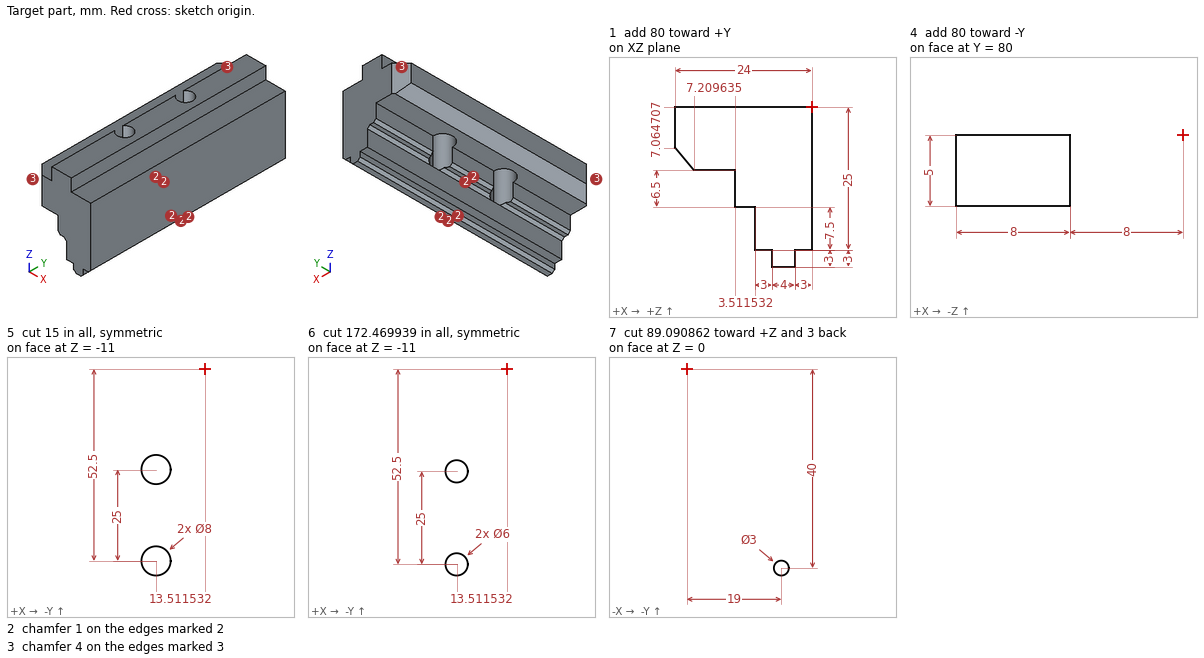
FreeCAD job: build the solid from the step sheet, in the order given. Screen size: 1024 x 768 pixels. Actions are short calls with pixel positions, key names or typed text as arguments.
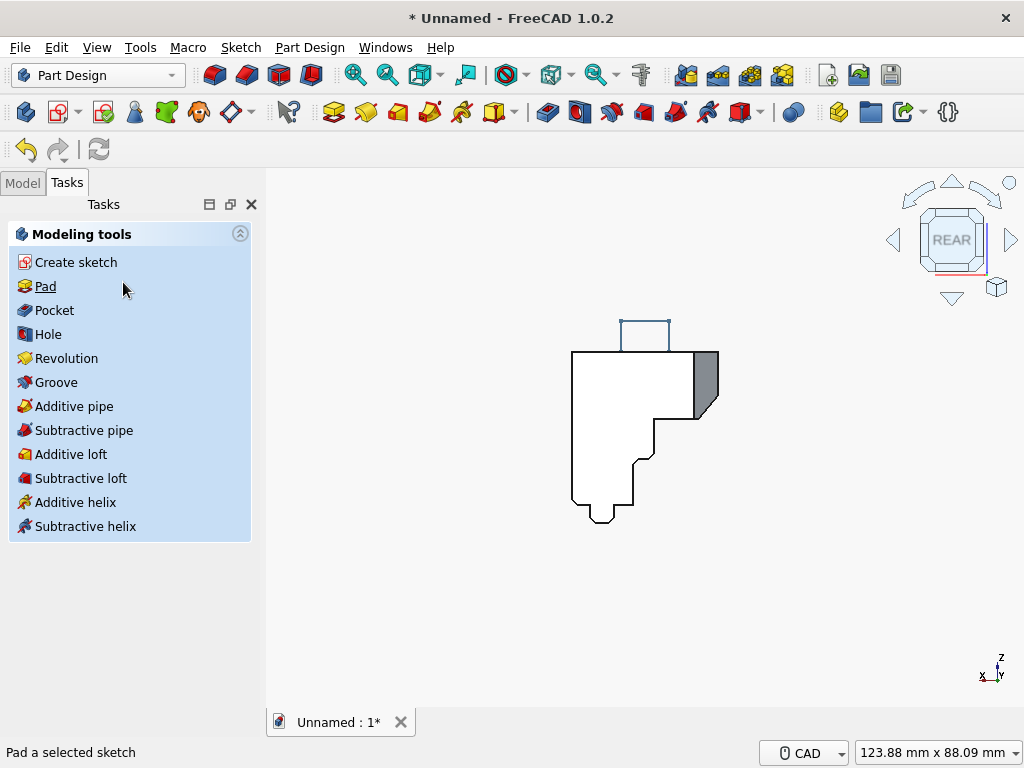
click(334, 112)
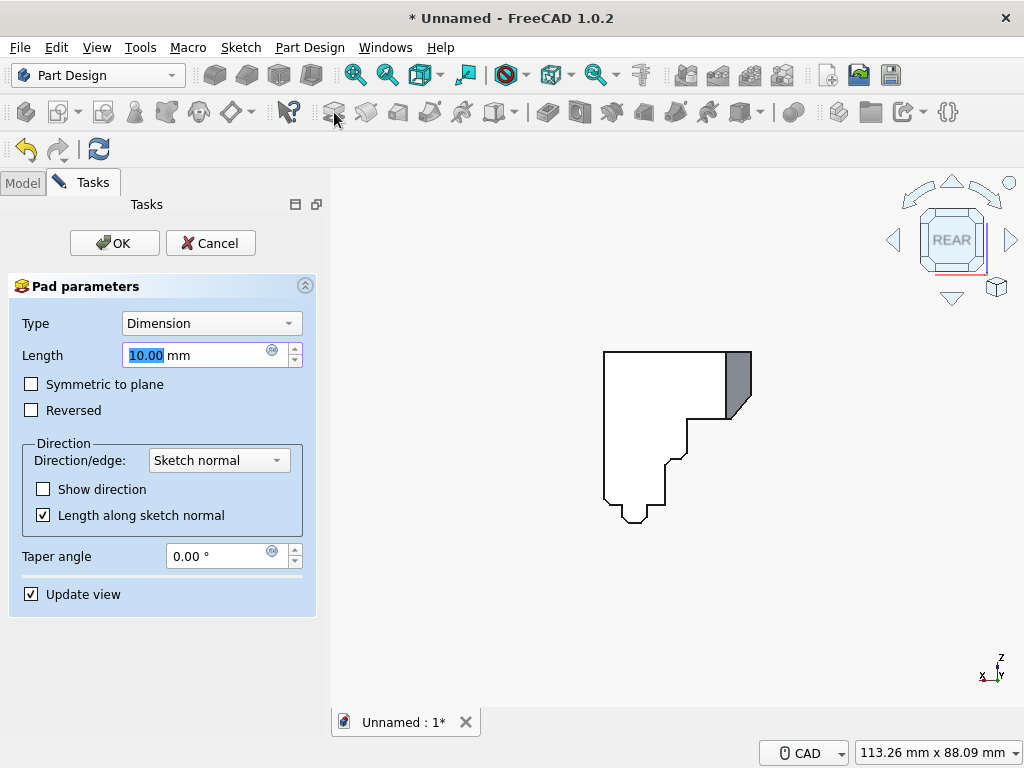
text(80)
key(Tab)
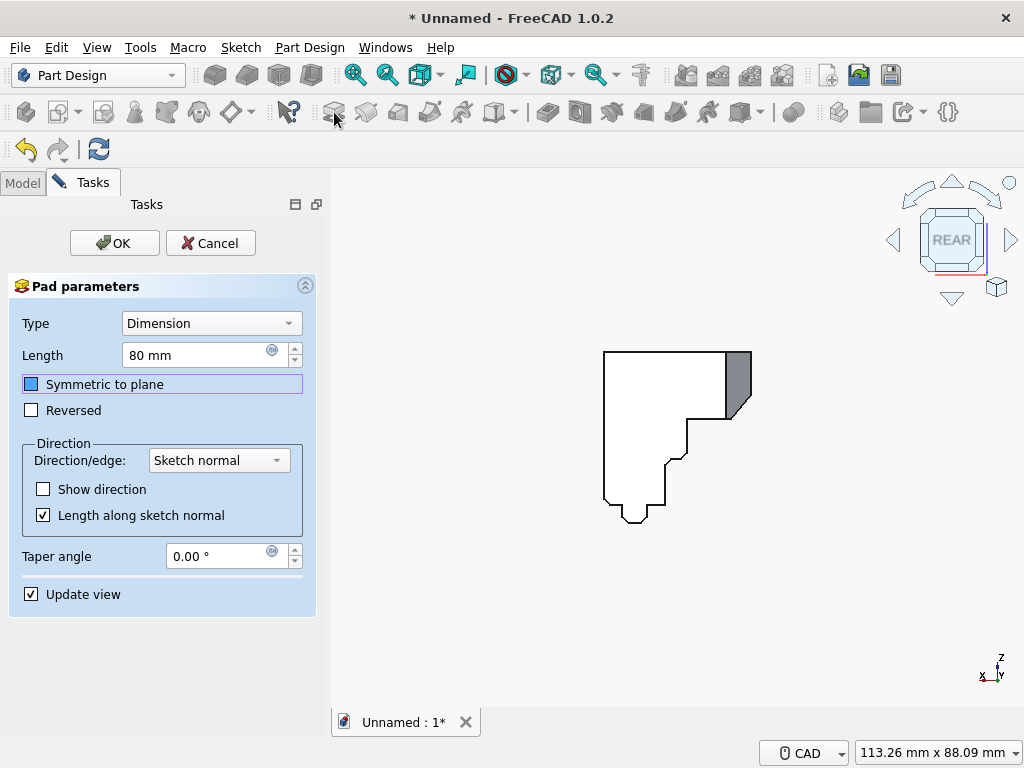
click(30, 410)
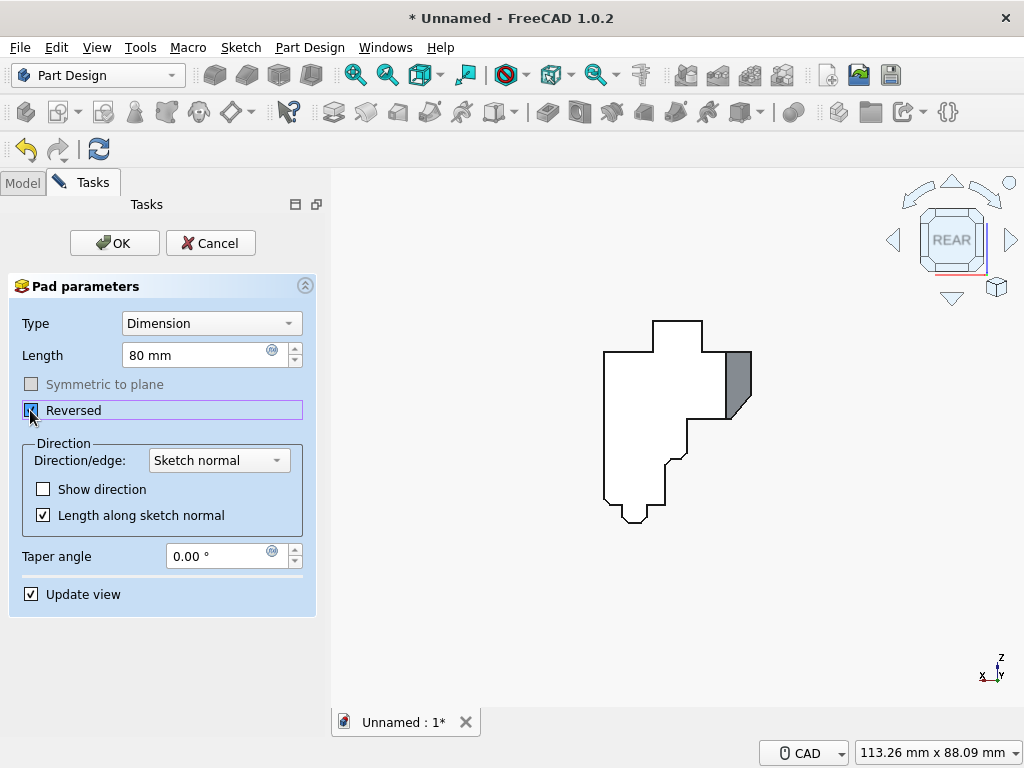
click(115, 243)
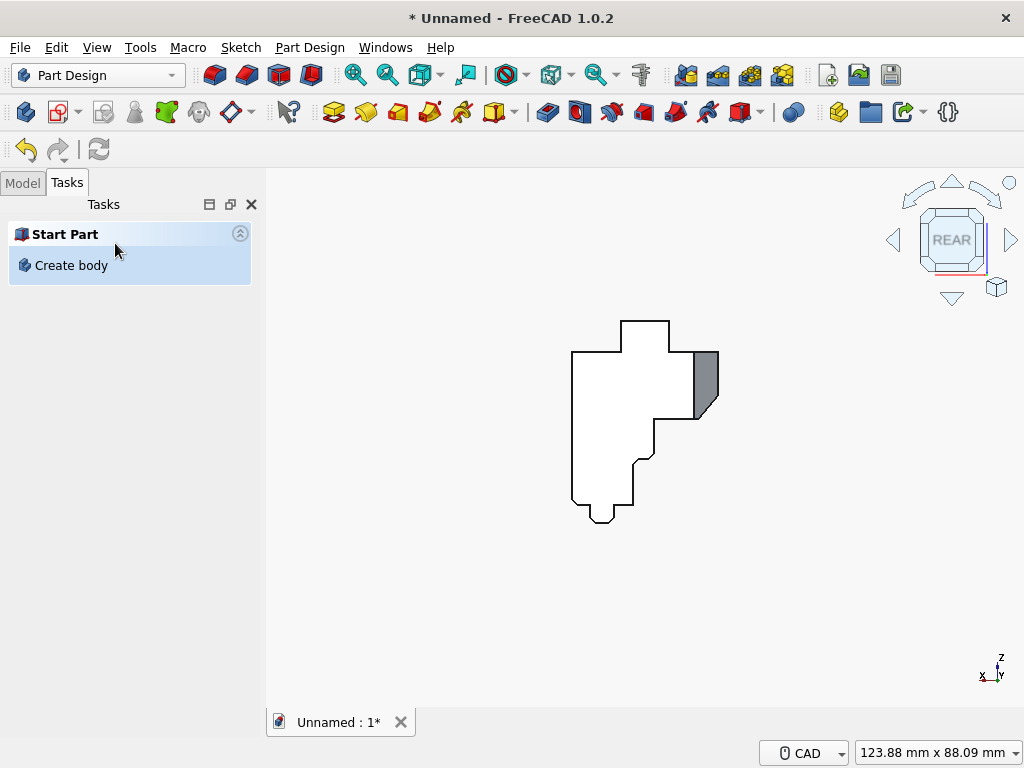
key(v)
key(f)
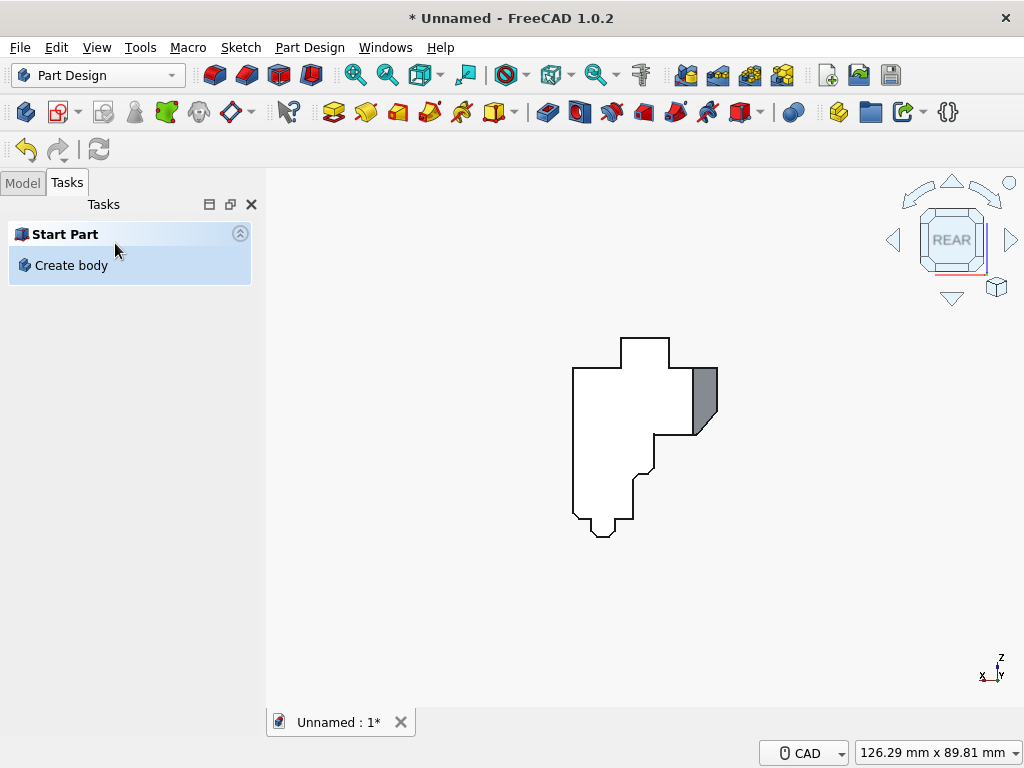
key(5)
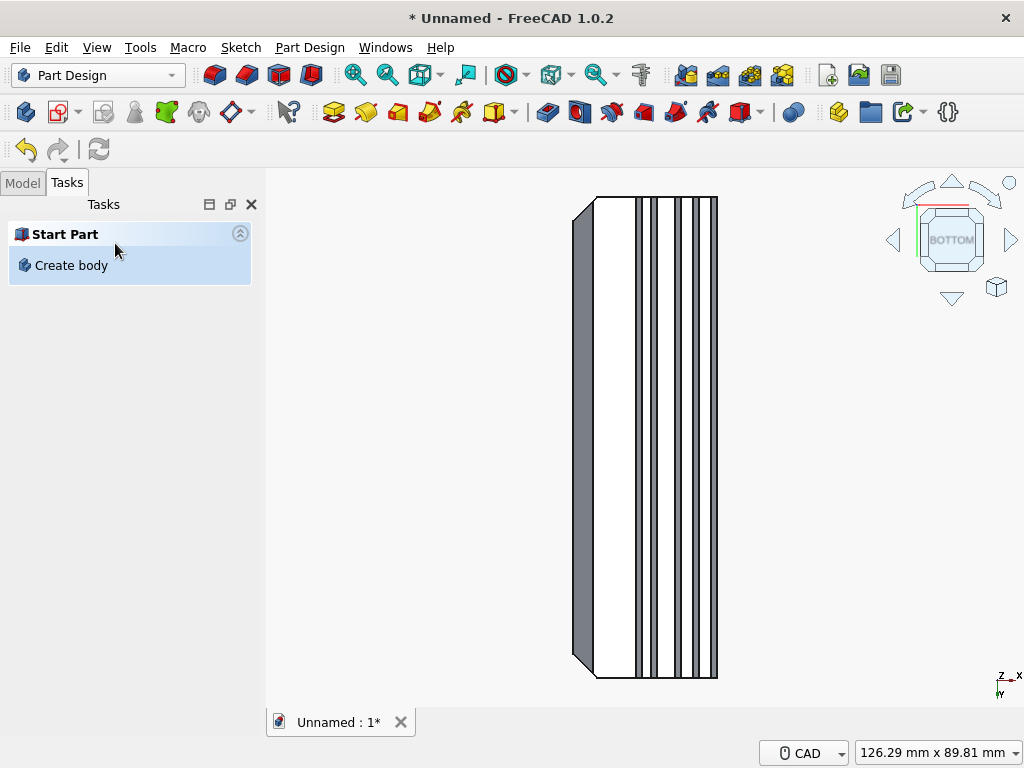
click(614, 642)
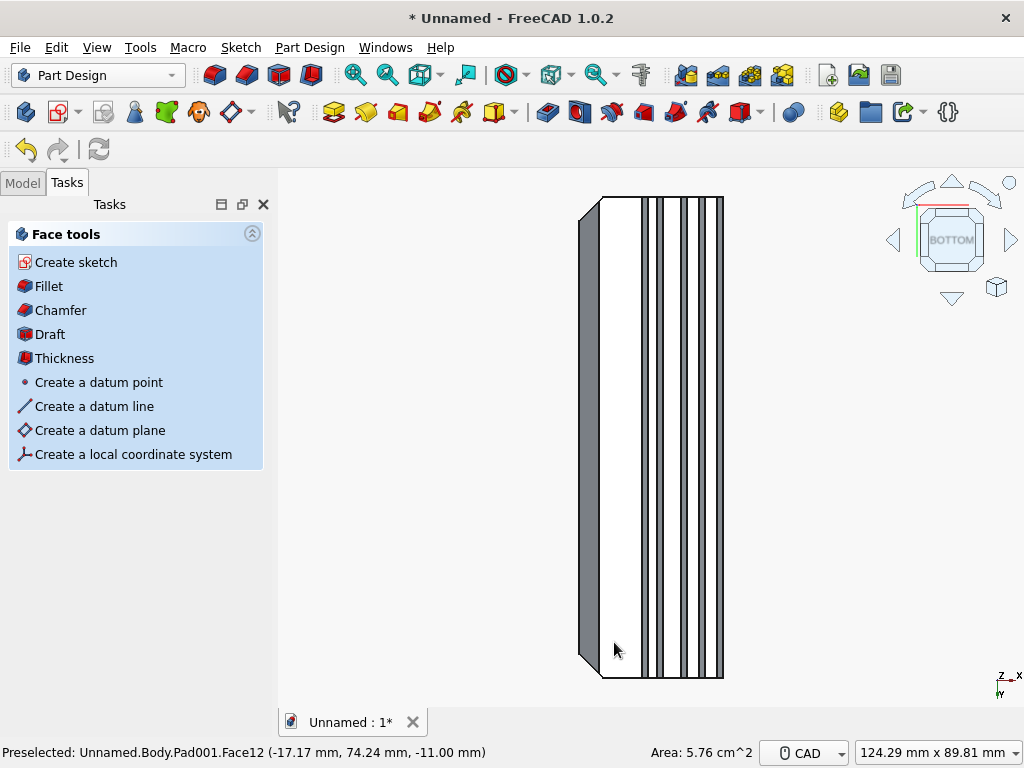
click(58, 112)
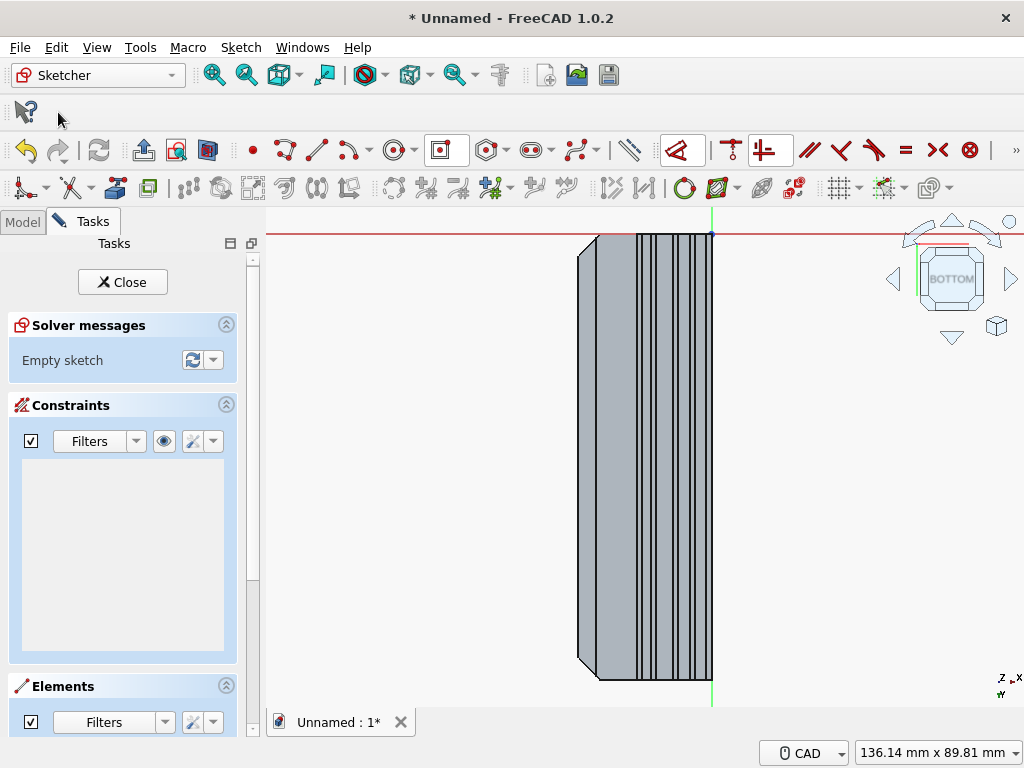
click(208, 150)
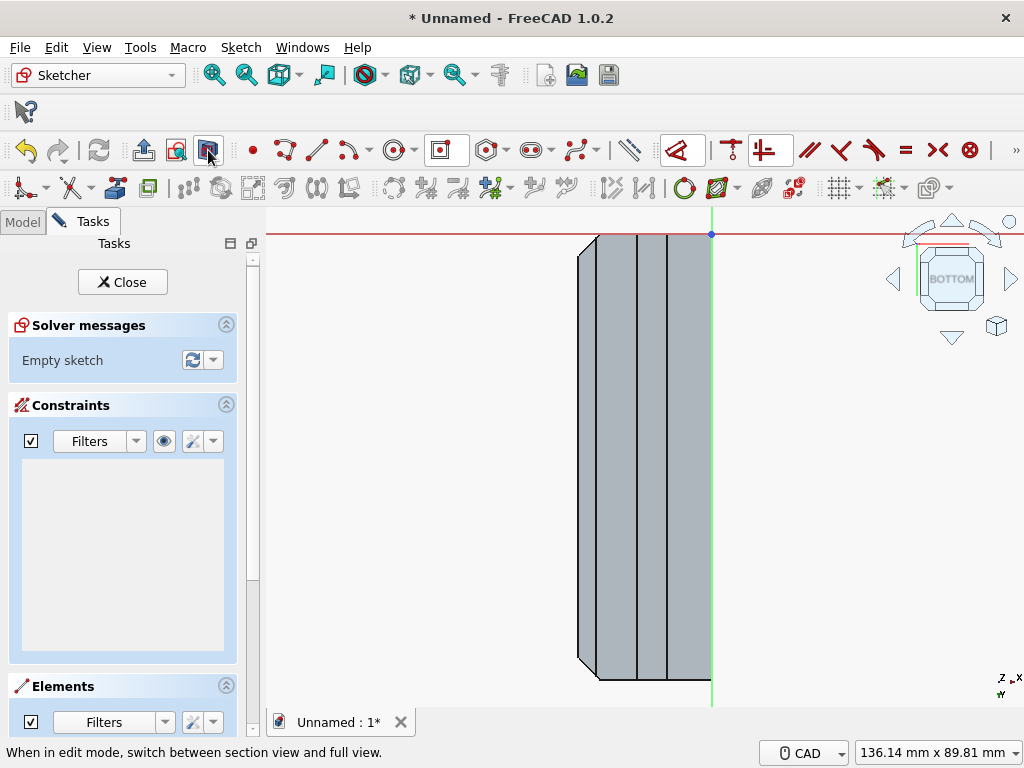
scroll(294, 679, down, 1)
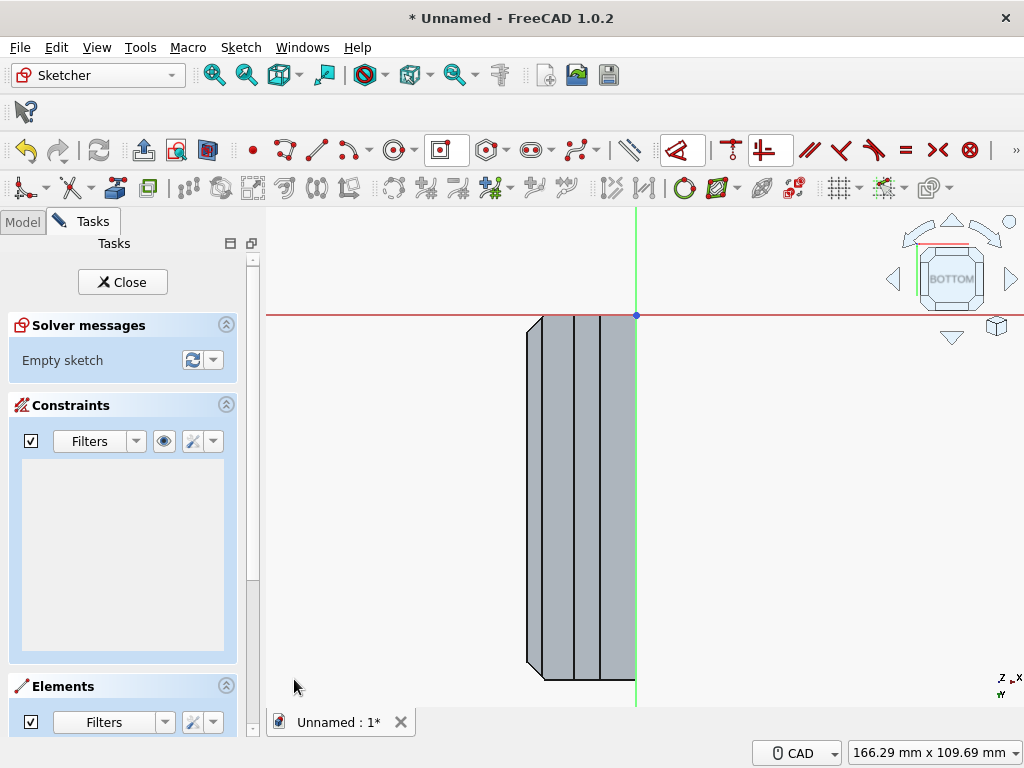
key(g)
key(c)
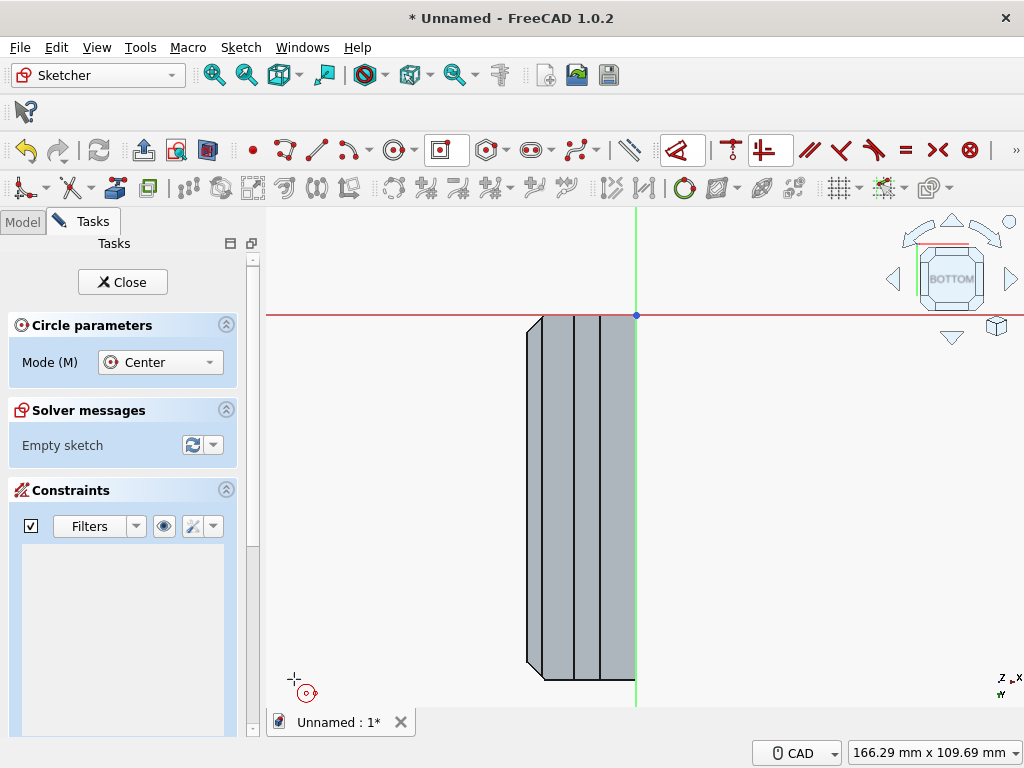
scroll(574, 554, up, 2)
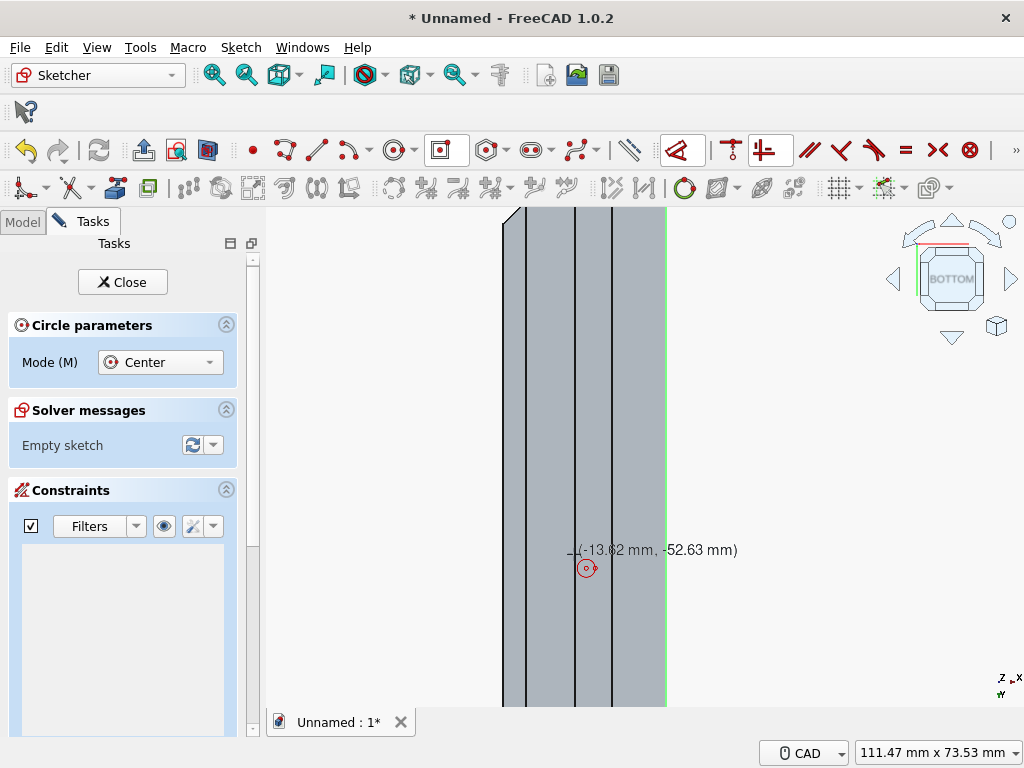
click(575, 554)
click(594, 535)